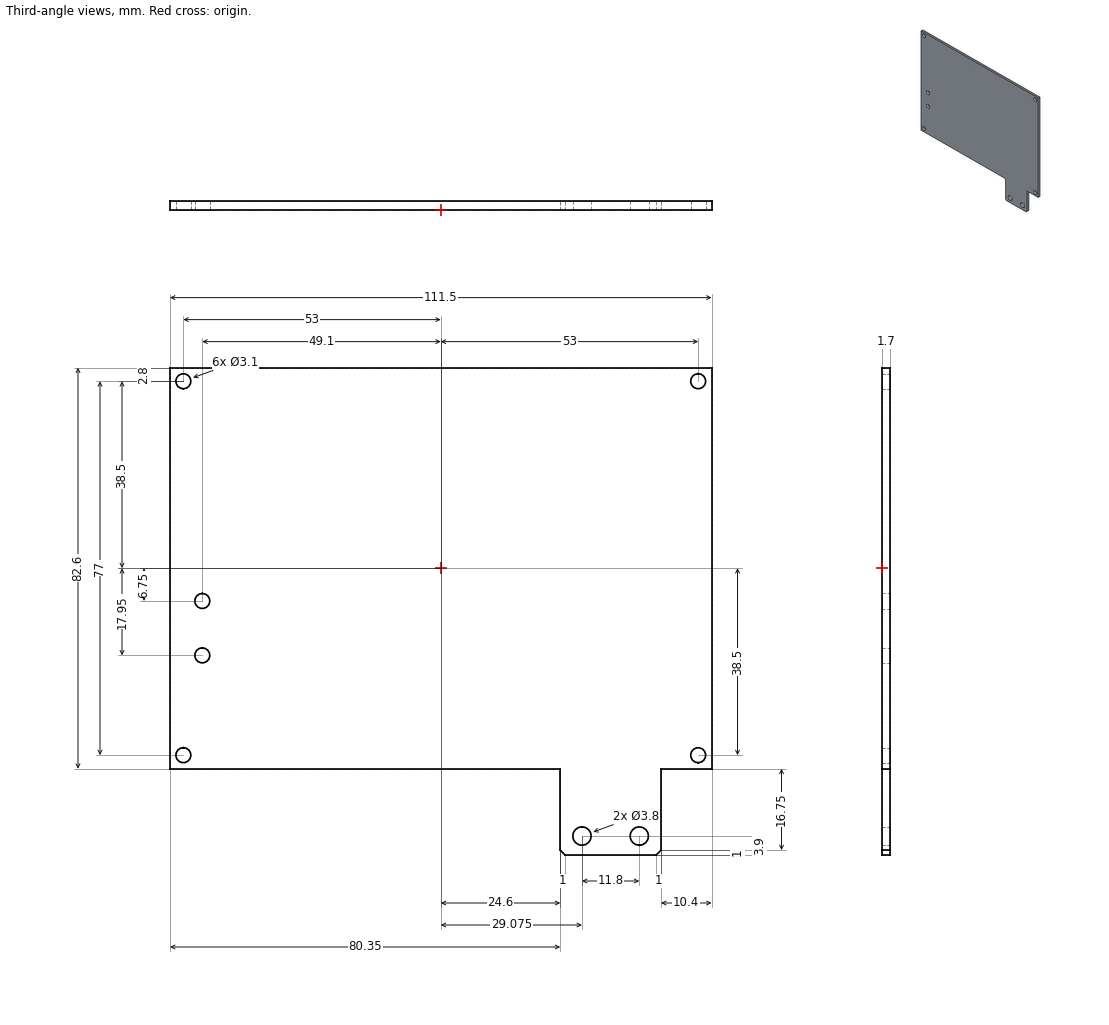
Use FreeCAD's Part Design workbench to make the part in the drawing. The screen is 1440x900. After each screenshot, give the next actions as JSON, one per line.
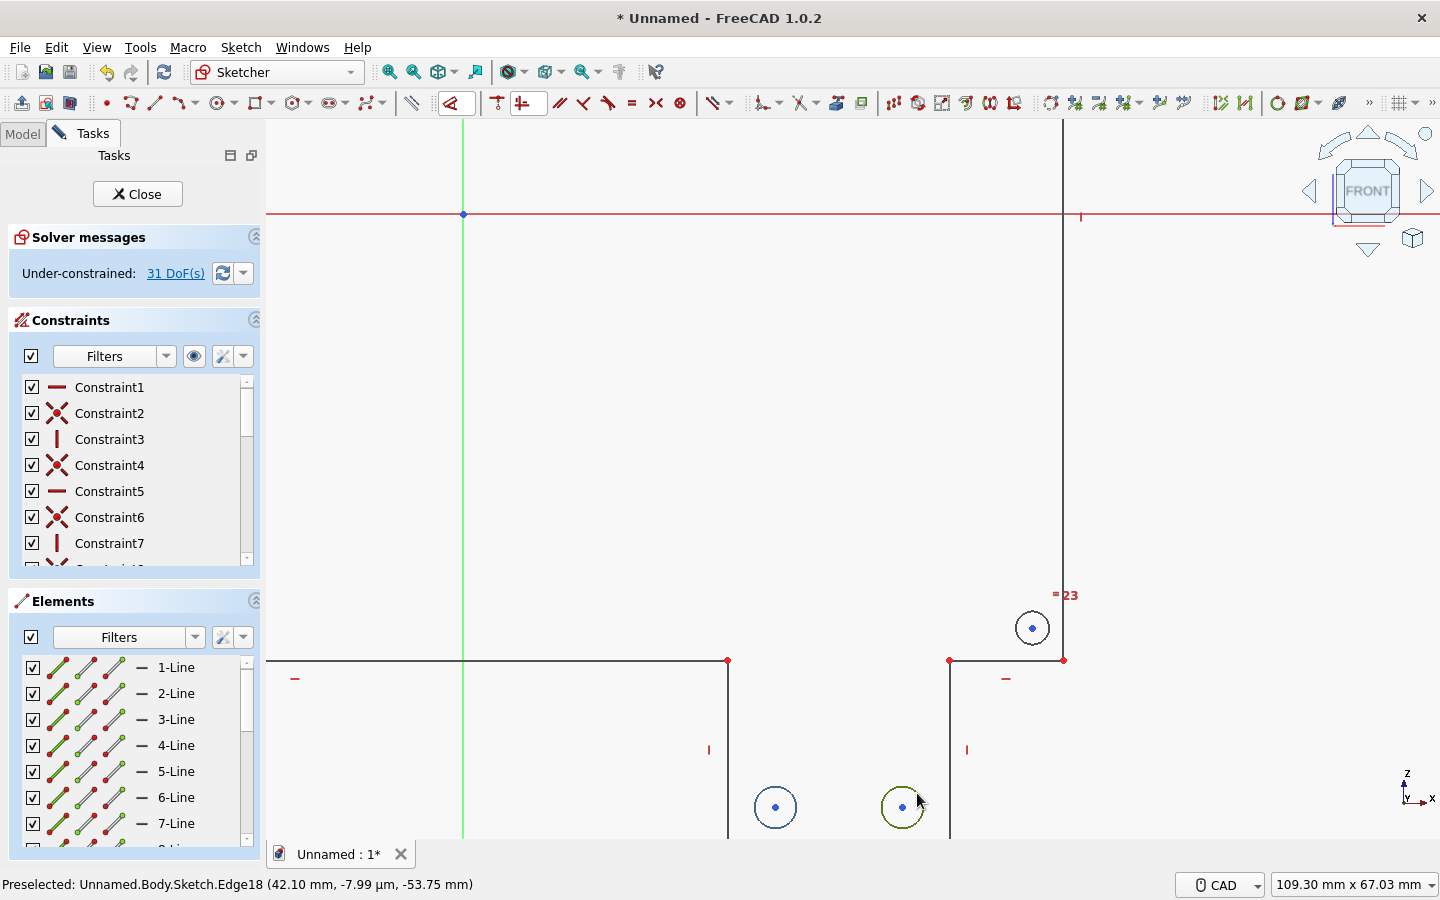
{"action": "left_click", "coordinate": [632, 104]}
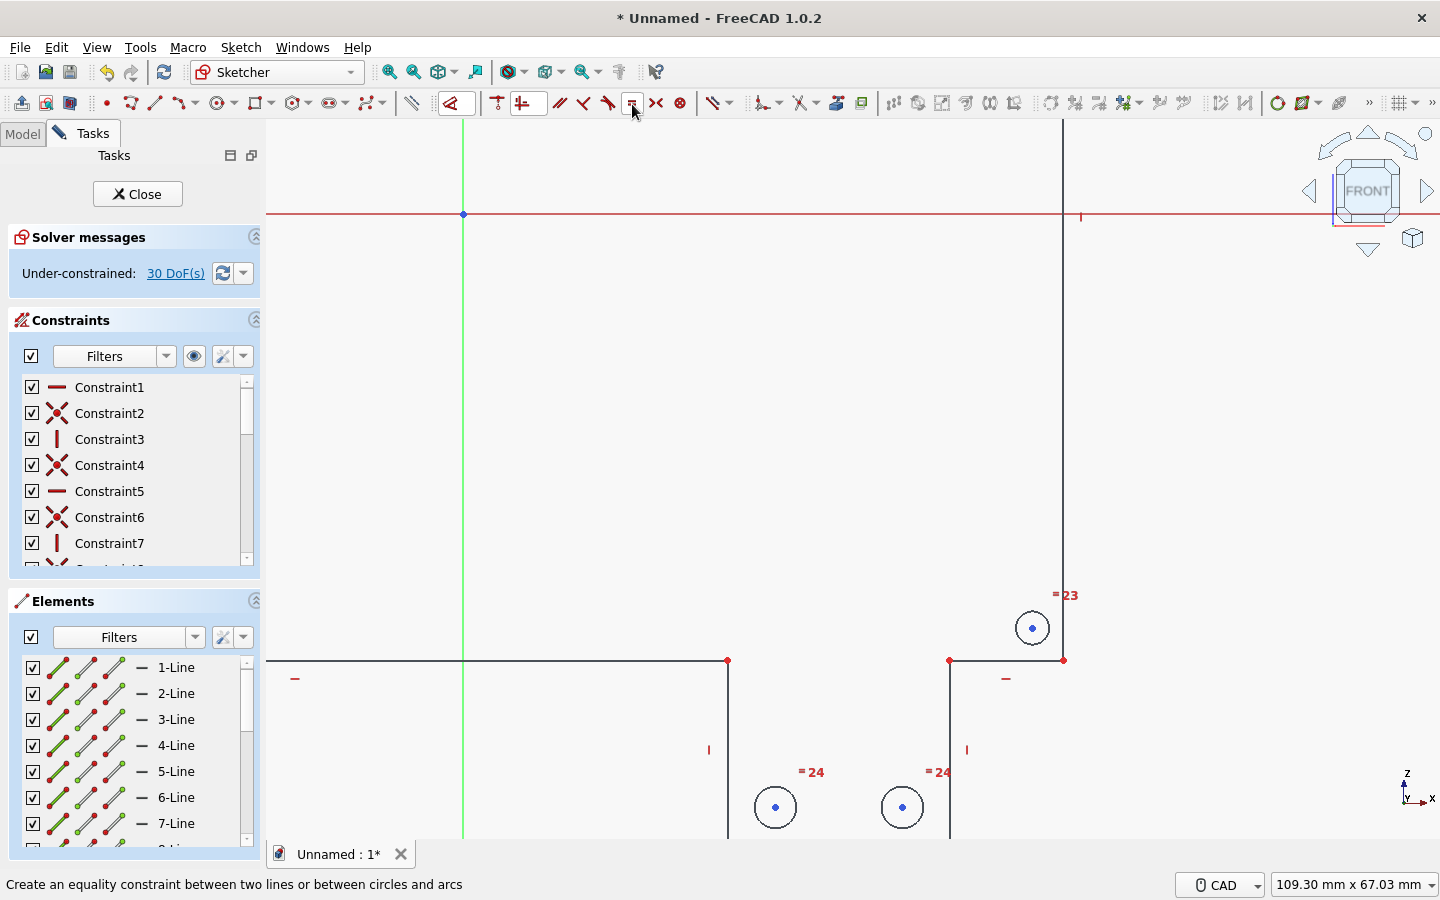
{"action": "scroll", "coordinate": [1046, 617], "scroll_direction": "down", "scroll_amount": 4}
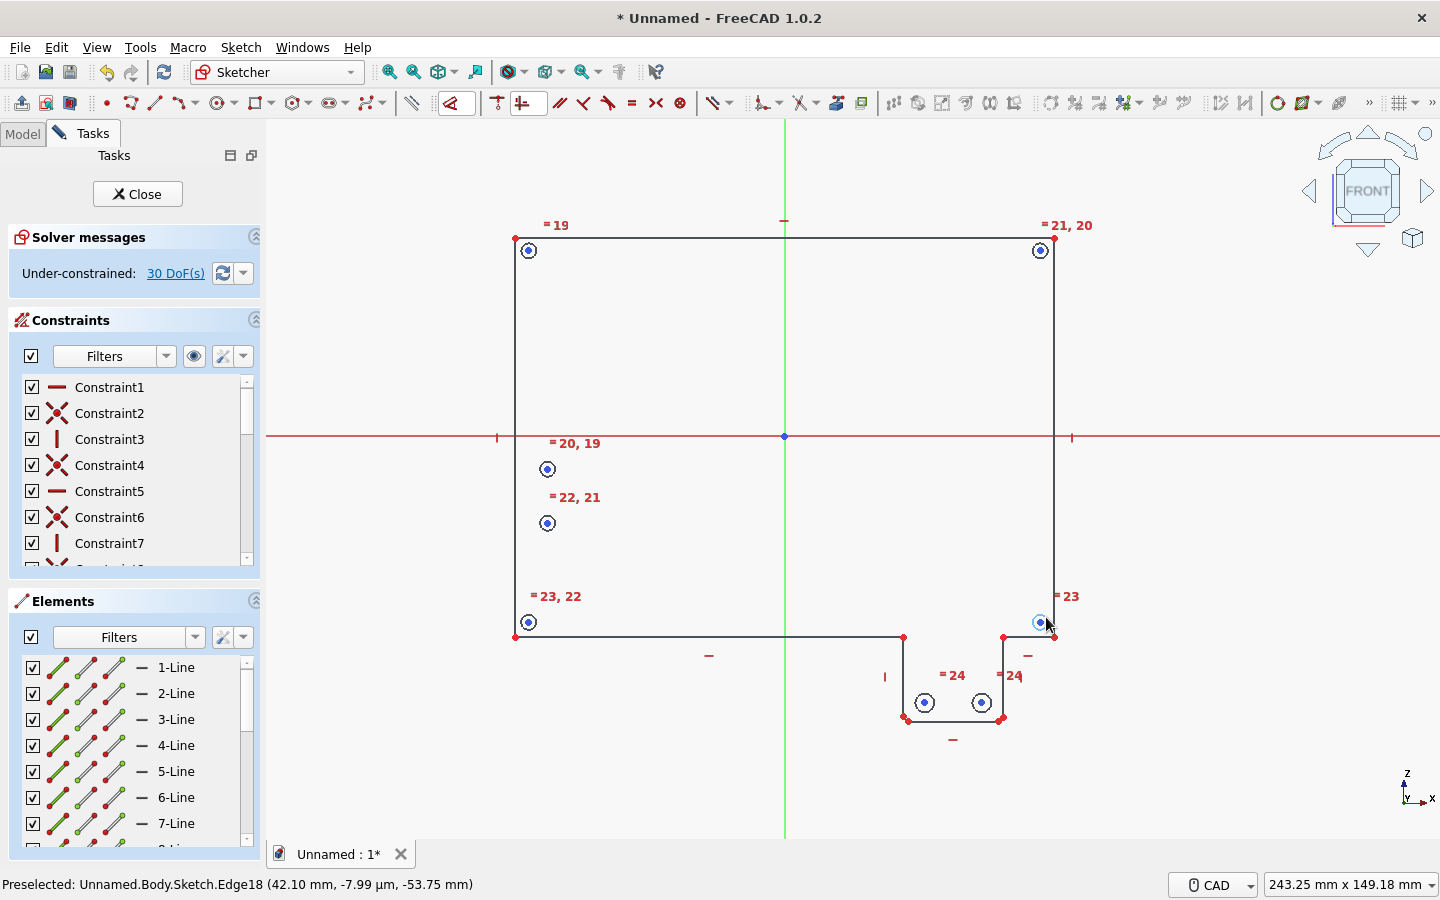
{"action": "left_click", "coordinate": [548, 469]}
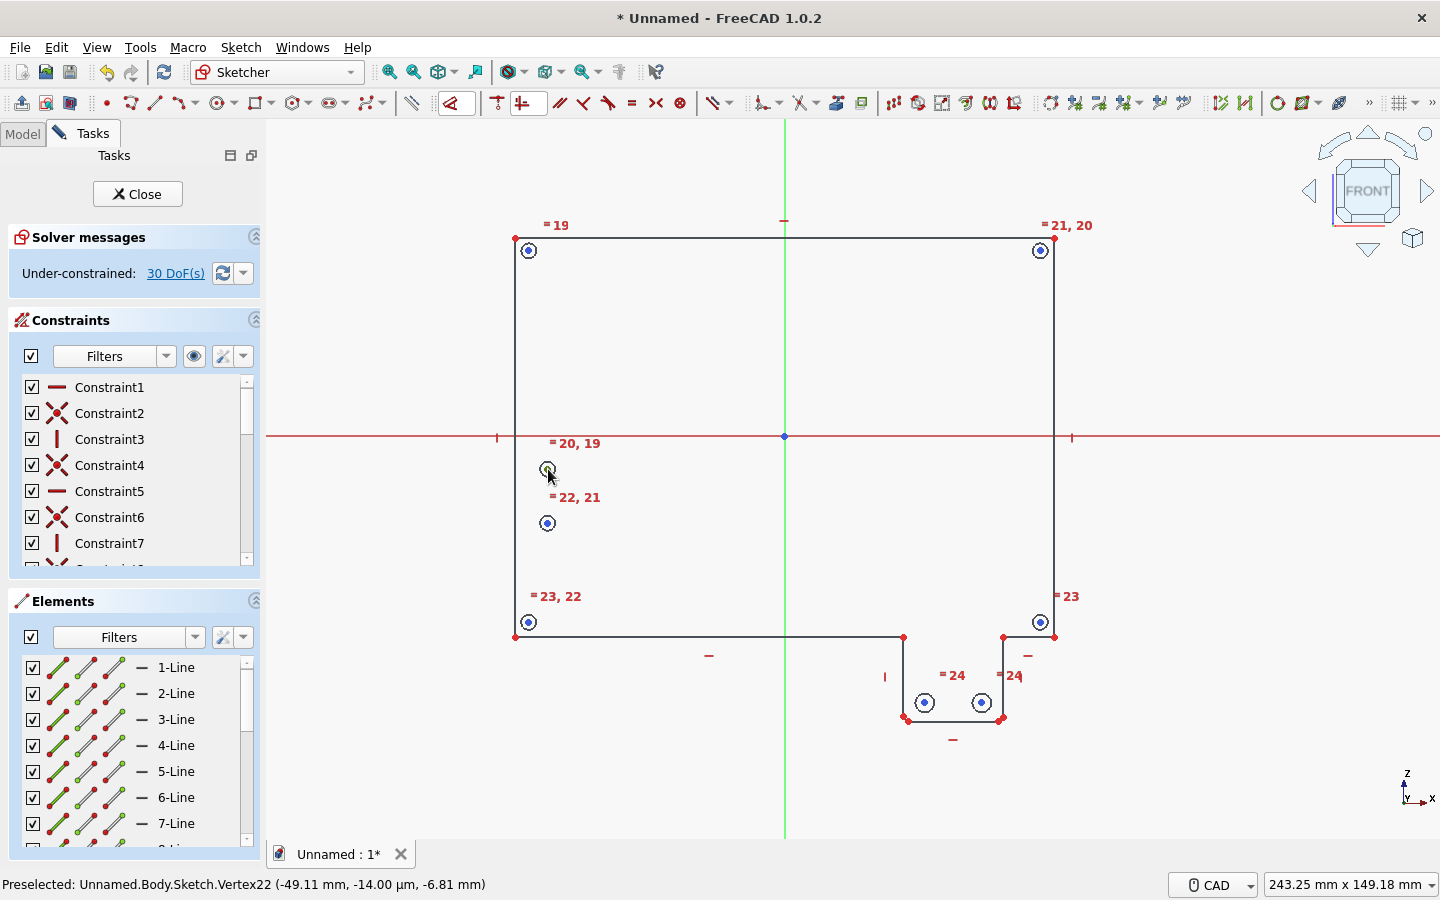
{"action": "left_click", "coordinate": [548, 523]}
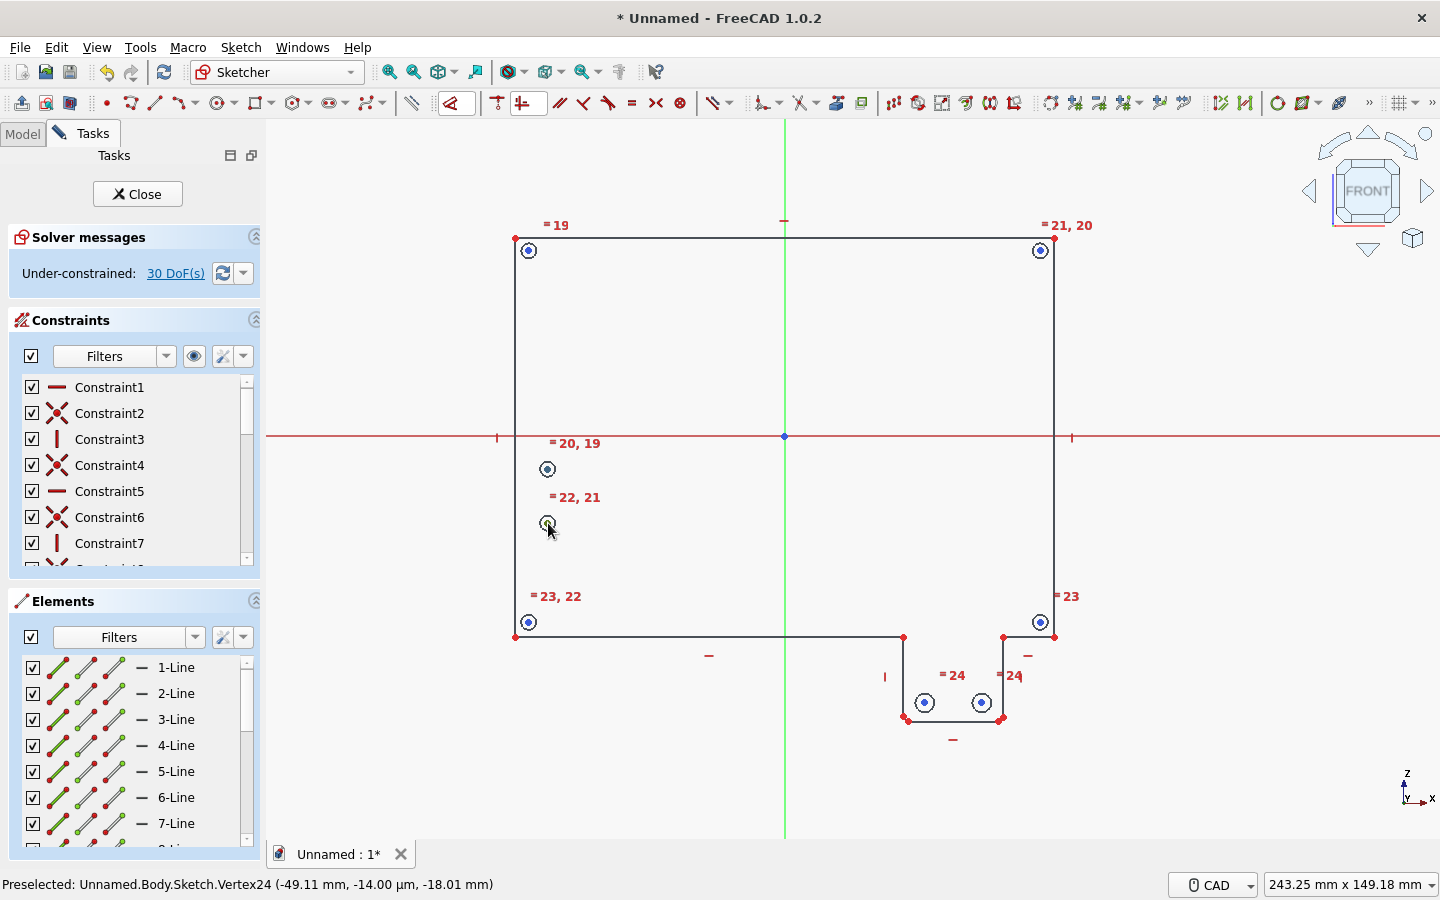
{"action": "key", "text": "v"}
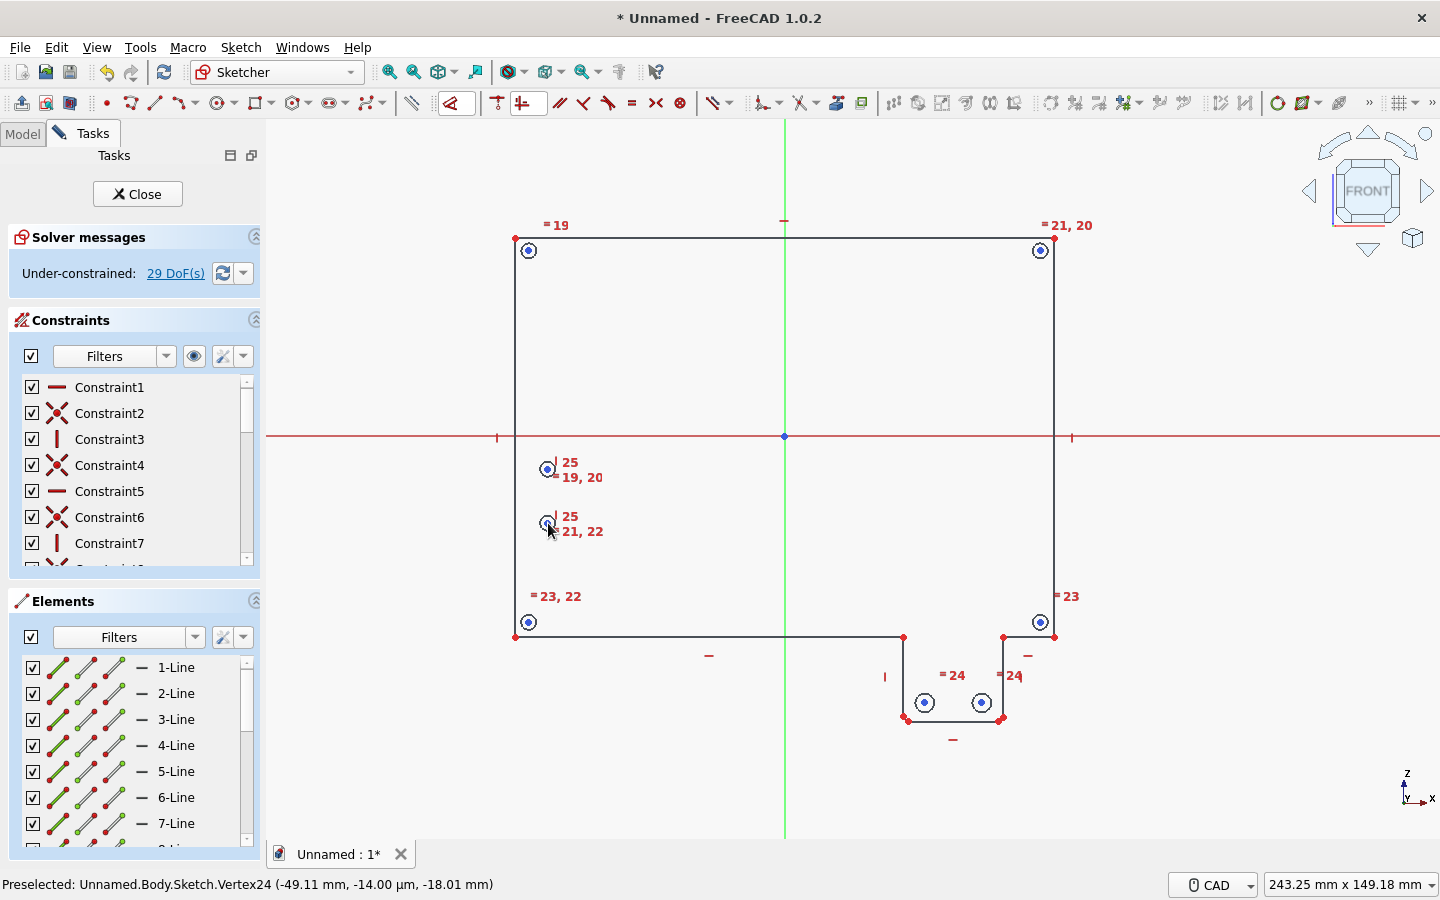
{"action": "left_click", "coordinate": [529, 251]}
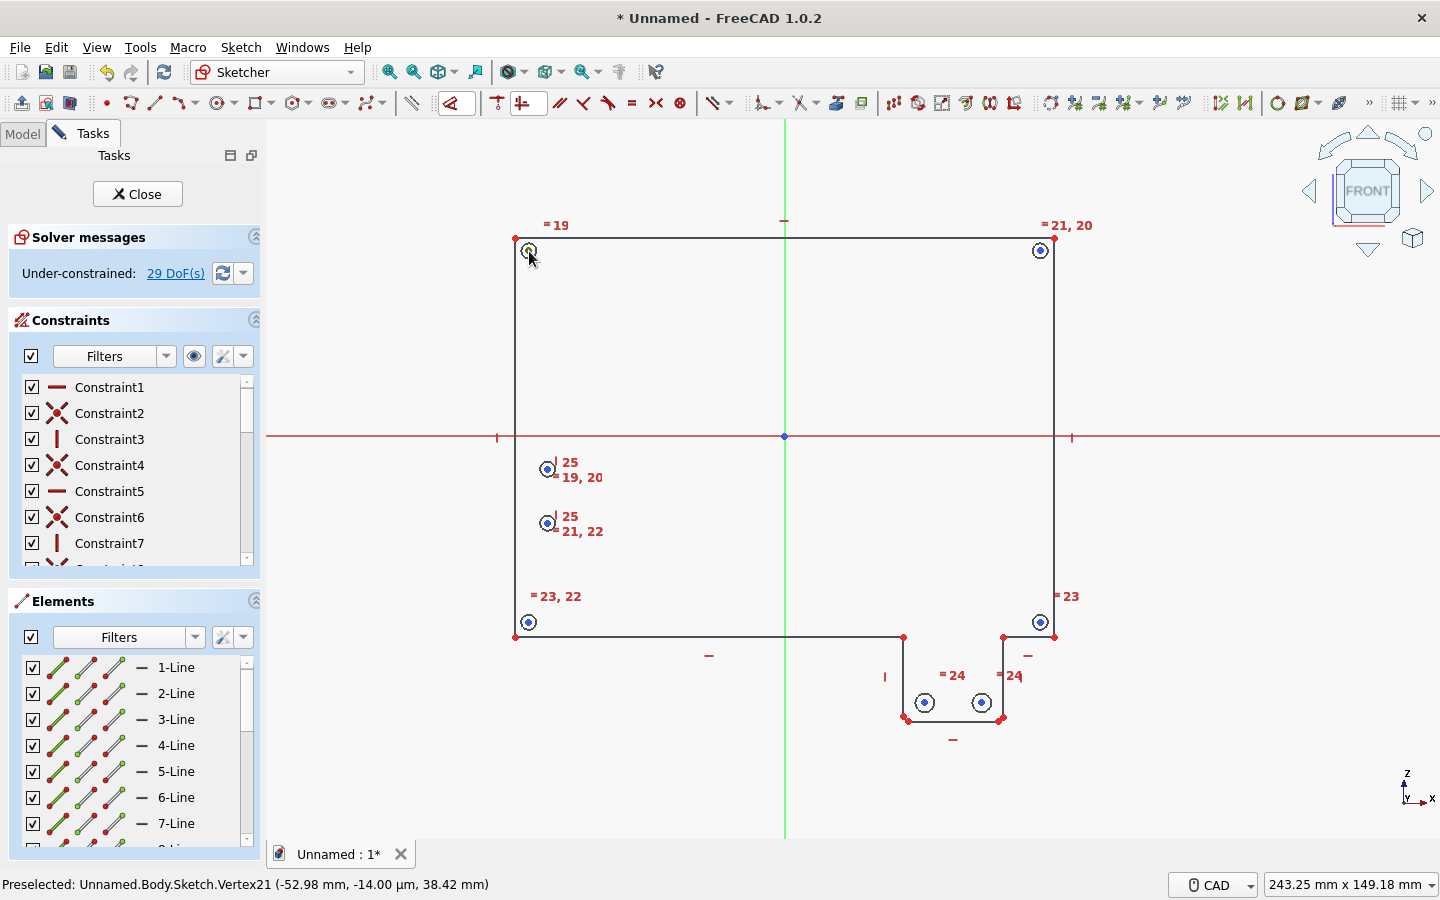
{"action": "left_click", "coordinate": [529, 622]}